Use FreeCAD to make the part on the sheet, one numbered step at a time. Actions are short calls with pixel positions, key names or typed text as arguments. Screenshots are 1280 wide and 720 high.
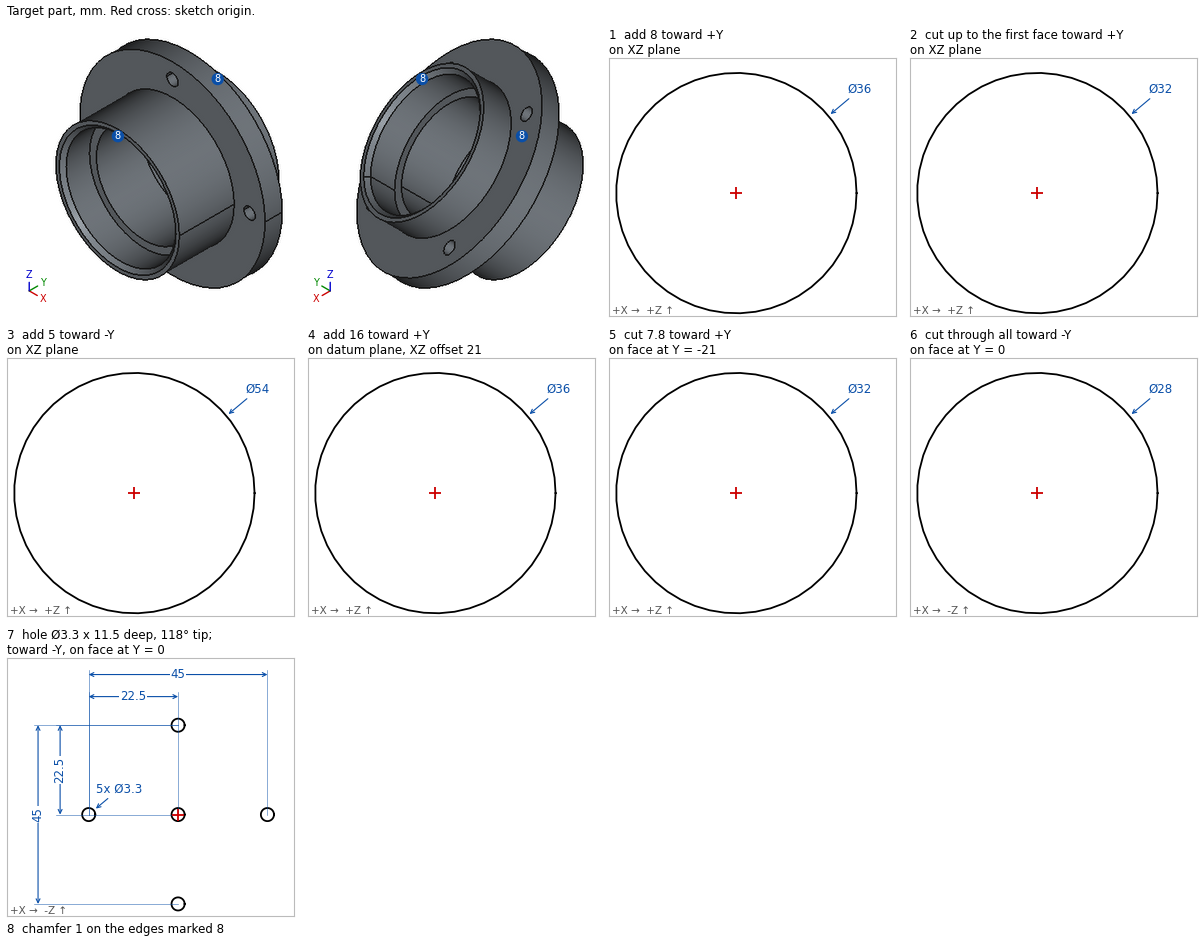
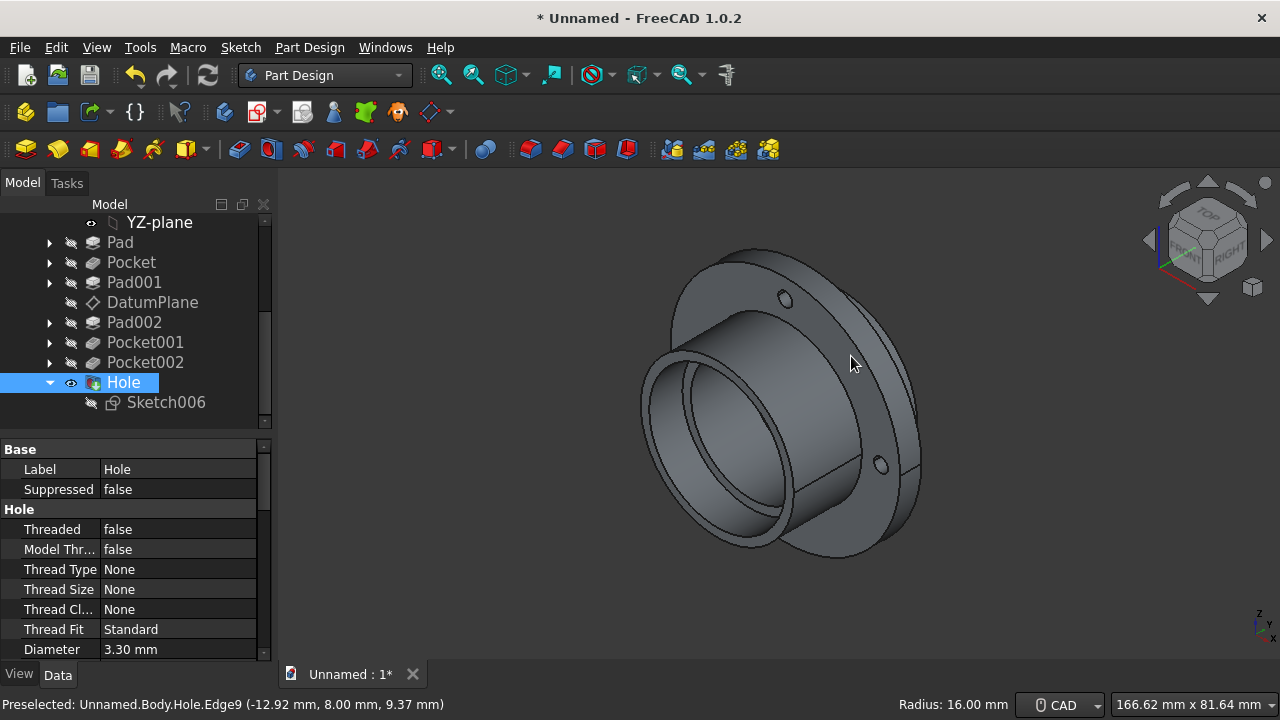
click(649, 409, ctrl)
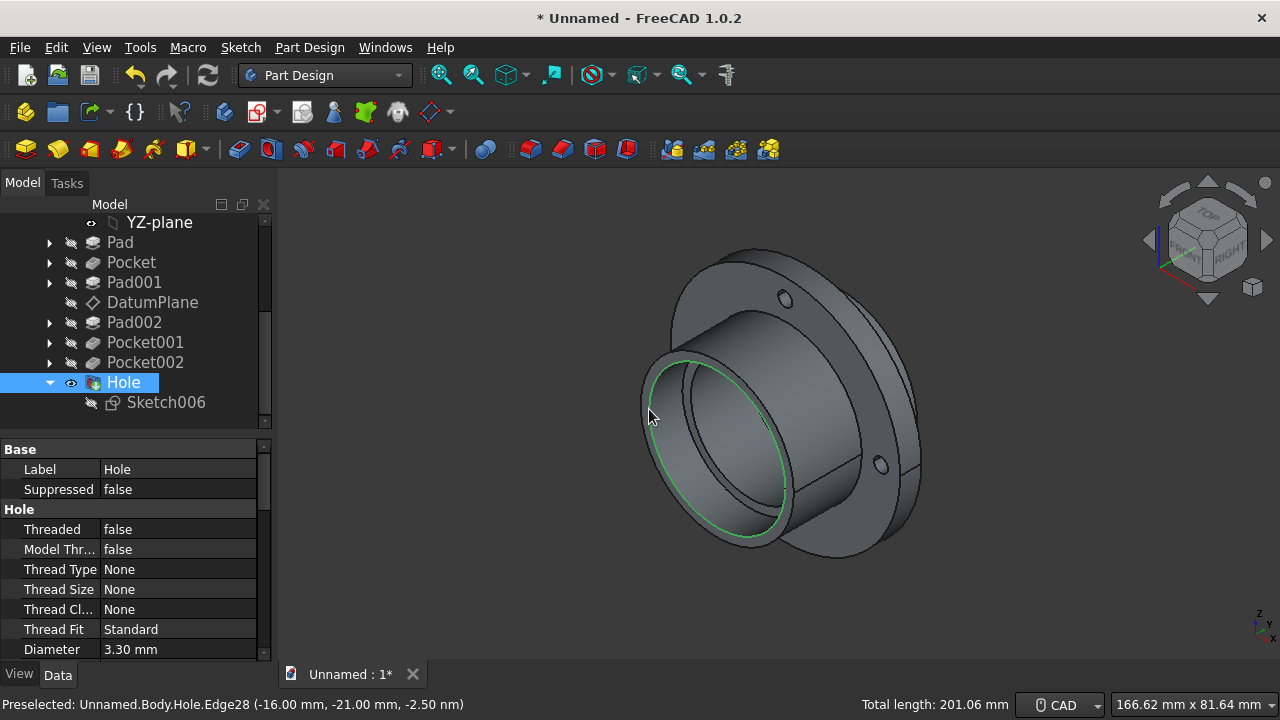
click(564, 150)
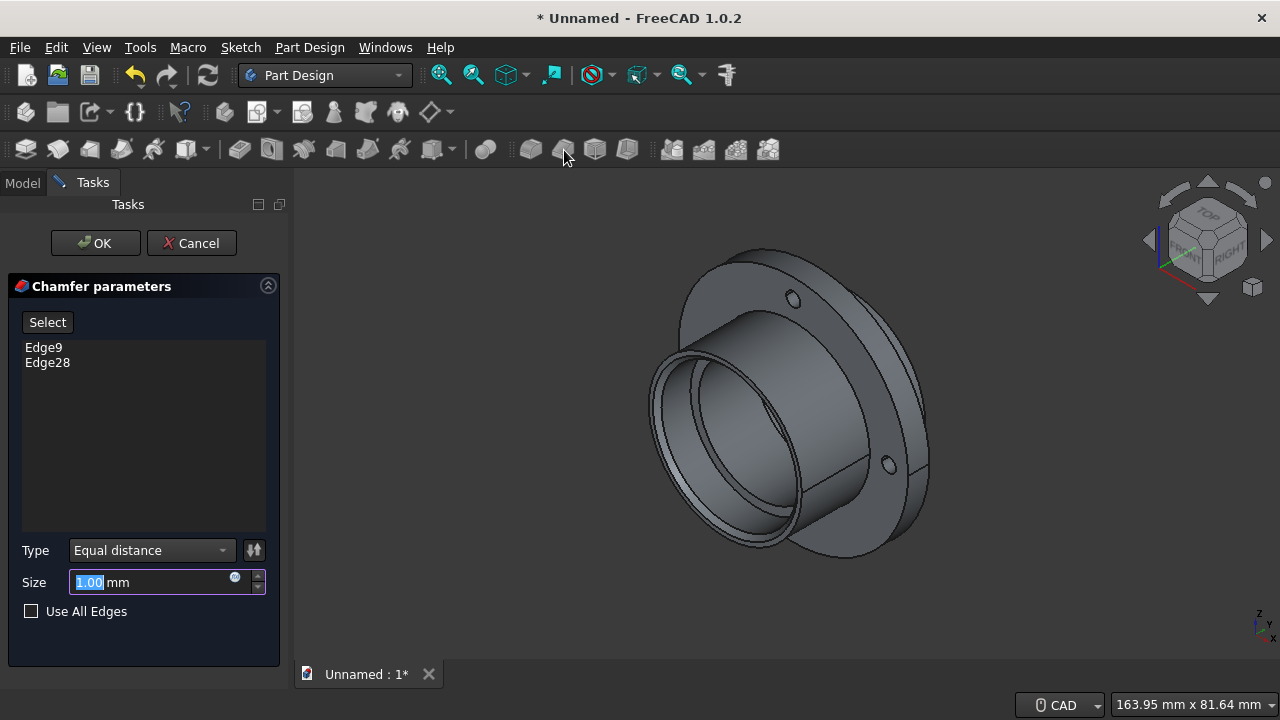
text(1)
key(Tab)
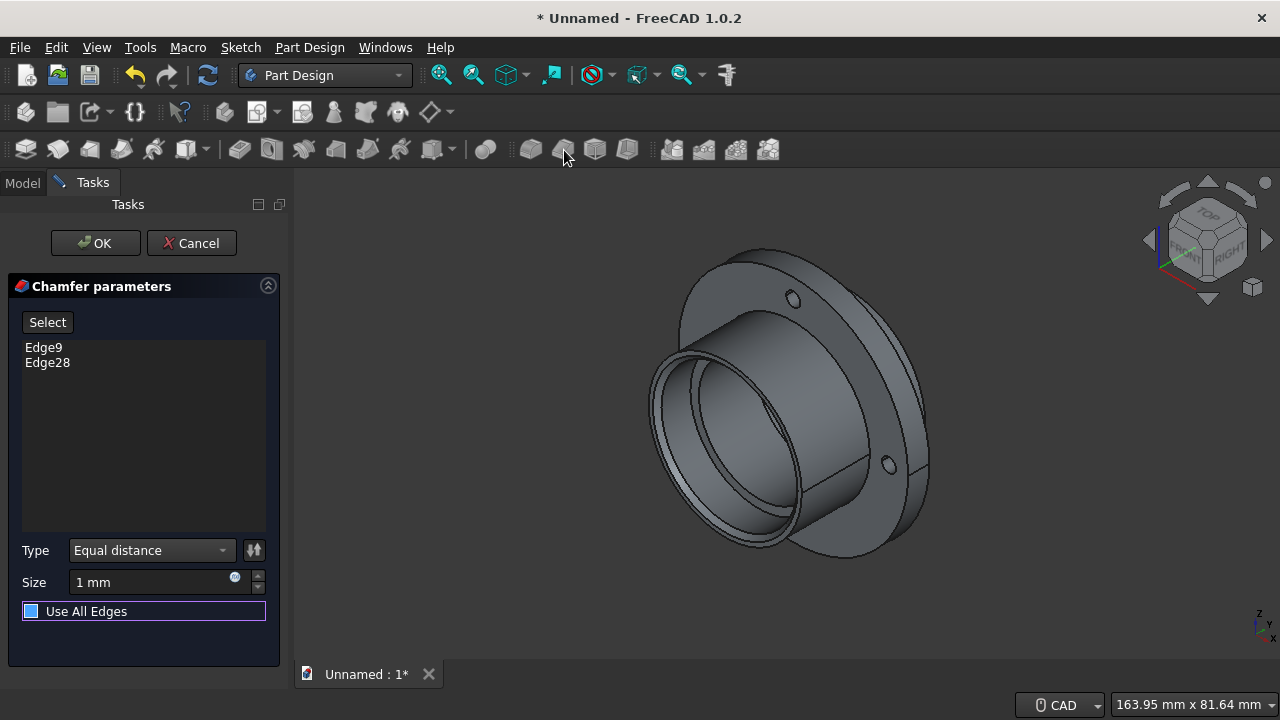
click(96, 243)